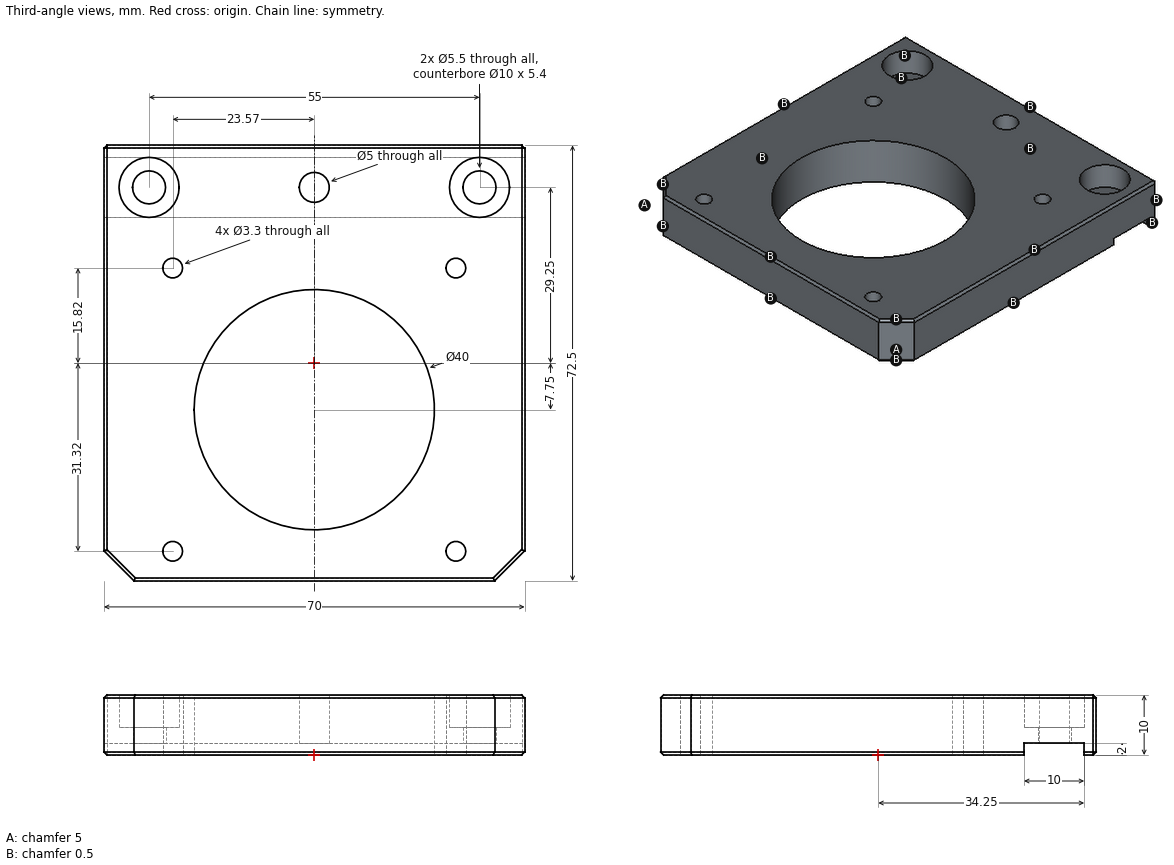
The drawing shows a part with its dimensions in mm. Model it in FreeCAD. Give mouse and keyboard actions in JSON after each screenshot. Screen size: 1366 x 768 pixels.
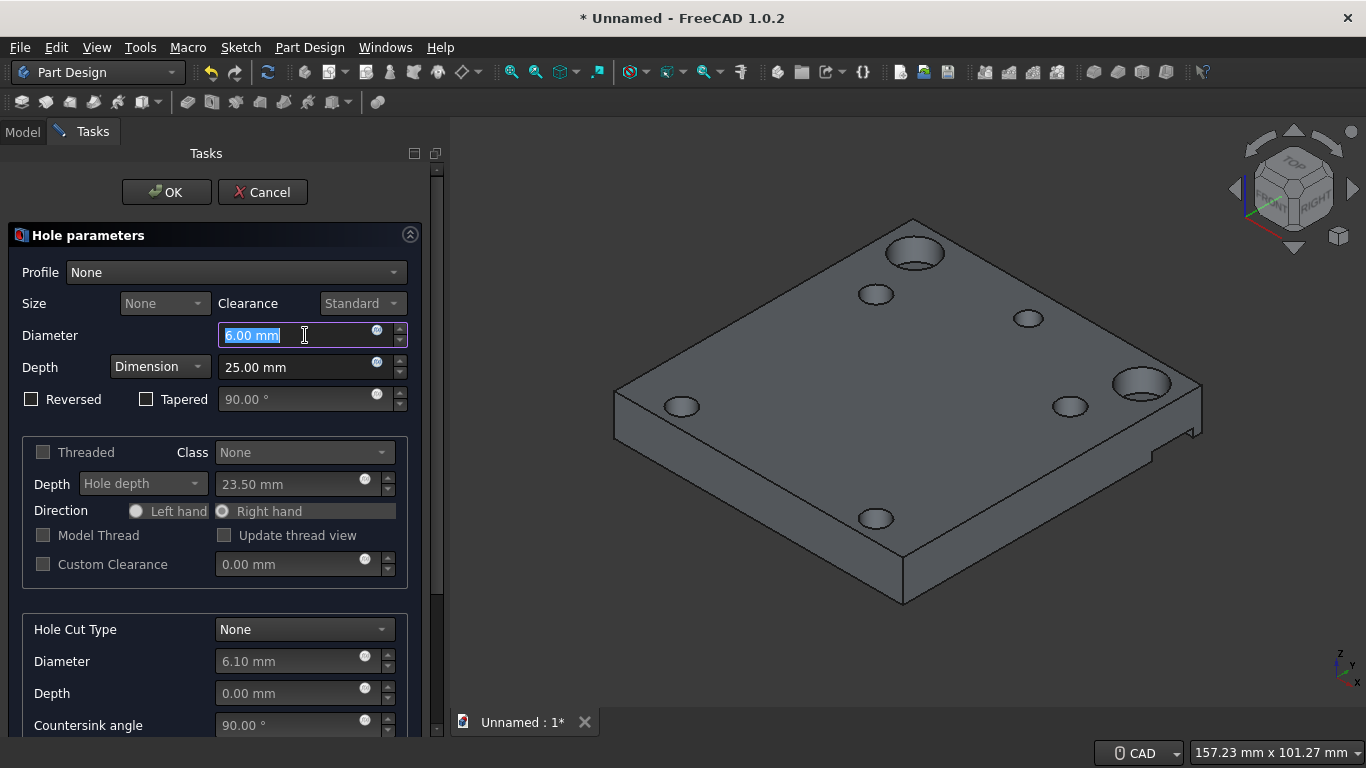
{"action": "type", "text": "3.3"}
{"action": "key", "text": "Tab"}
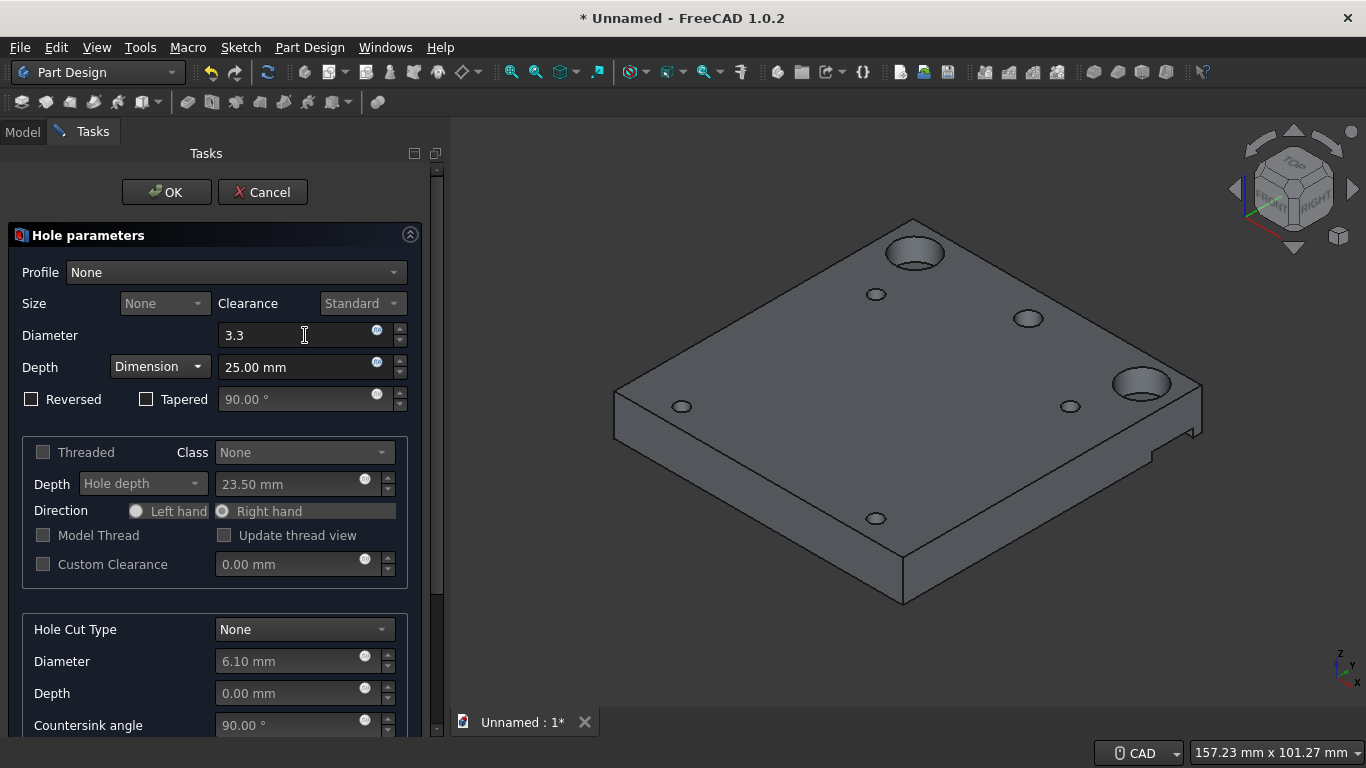
{"action": "left_click", "coordinate": [161, 366]}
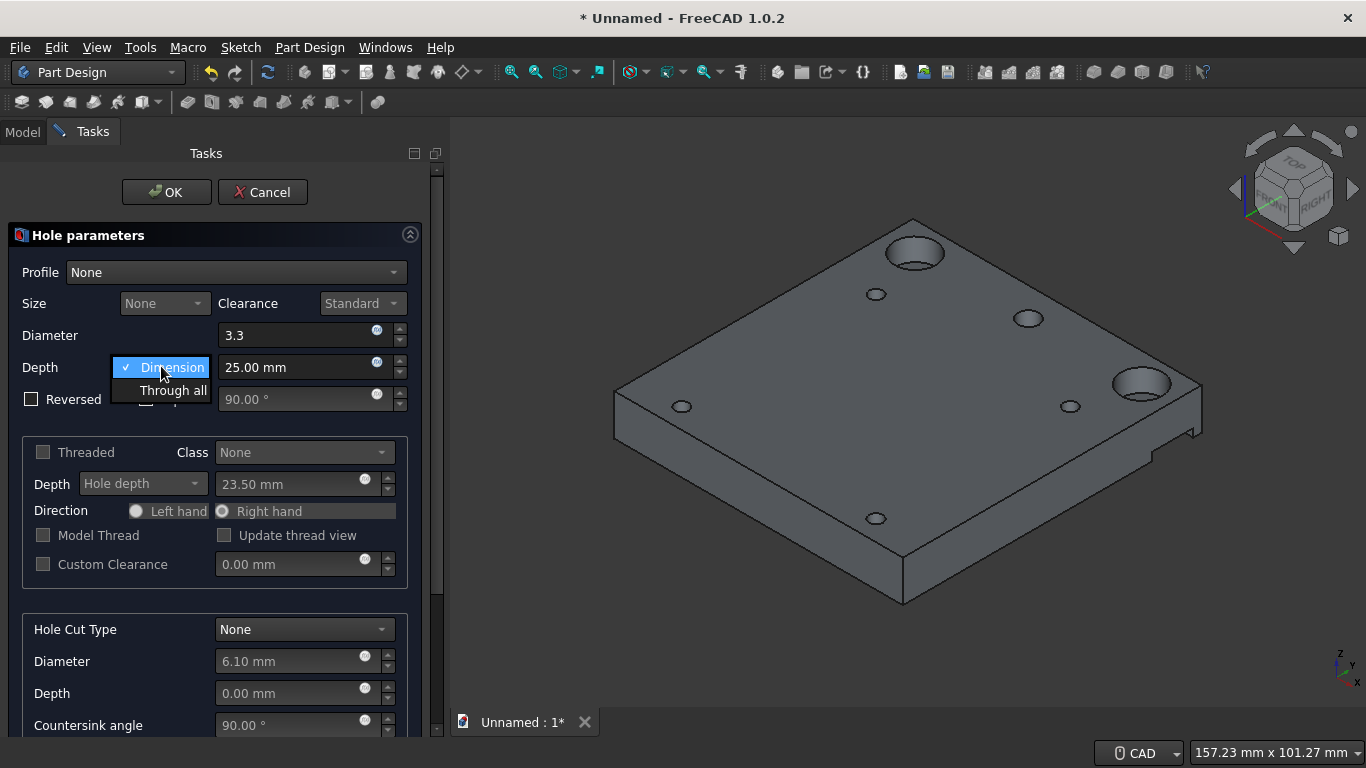
{"action": "left_click", "coordinate": [160, 390]}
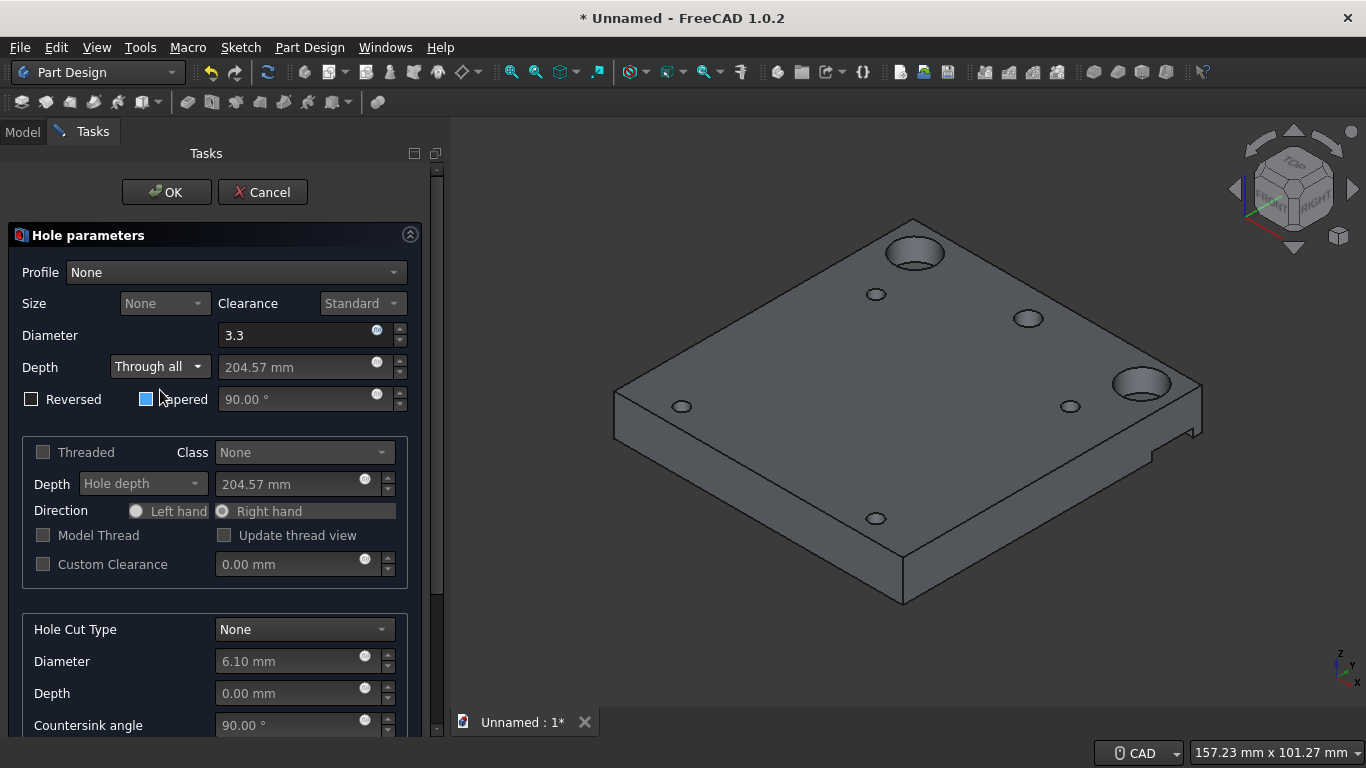
{"action": "left_click", "coordinate": [167, 192]}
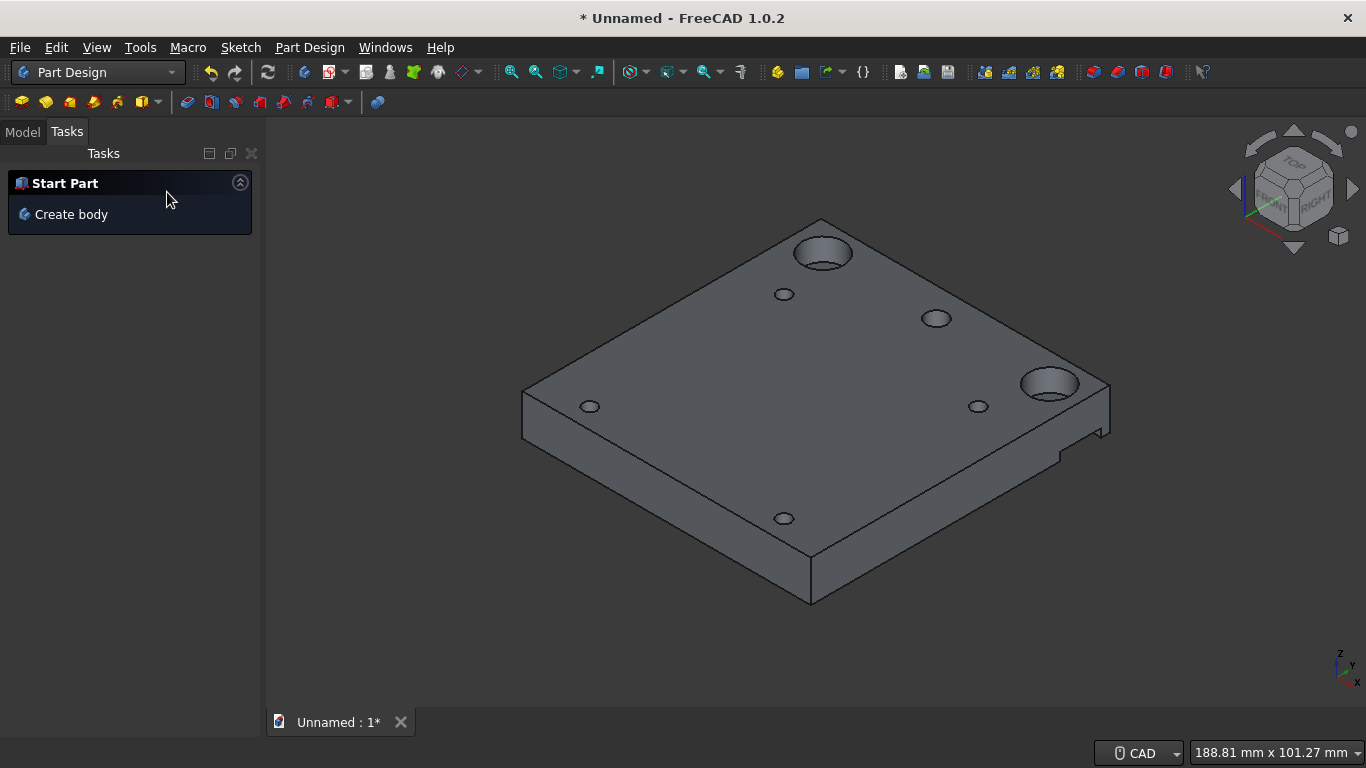
{"action": "left_click", "coordinate": [330, 72]}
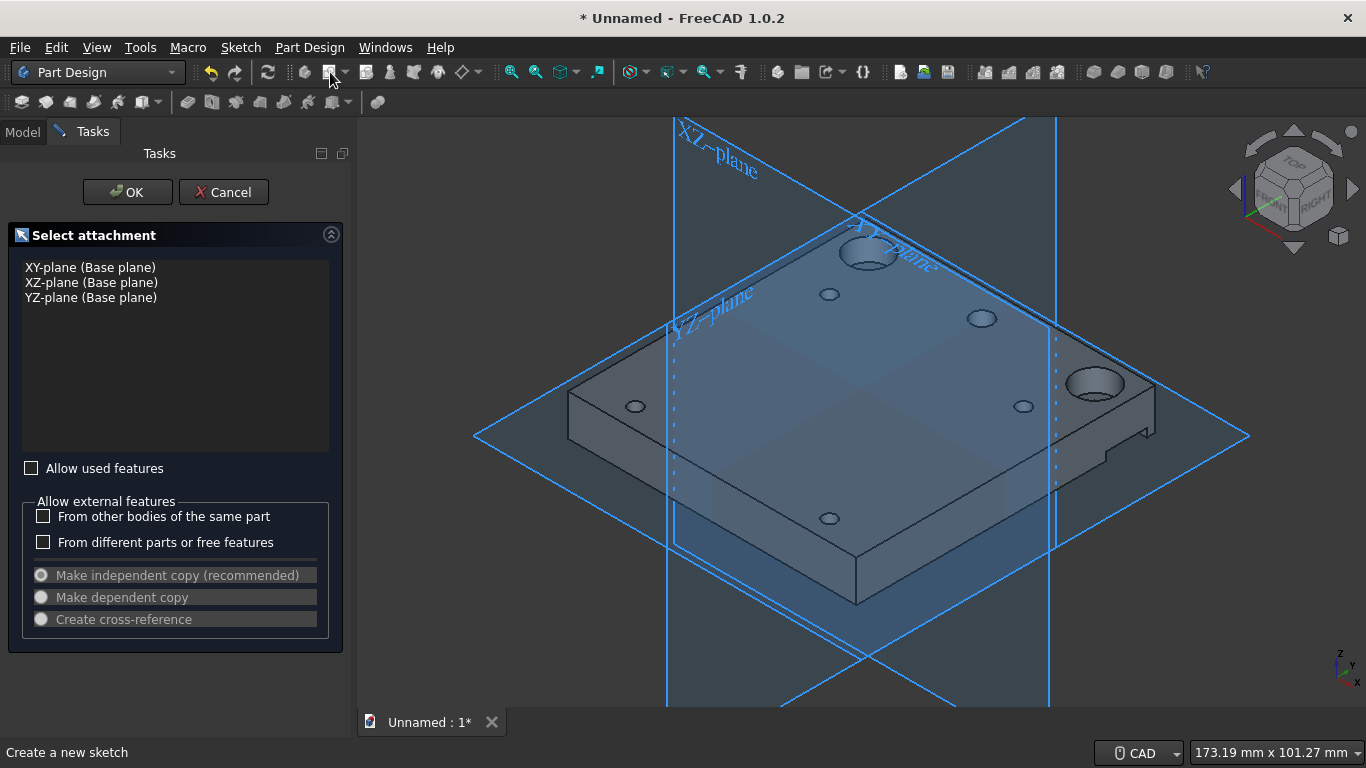
{"action": "left_click", "coordinate": [82, 268]}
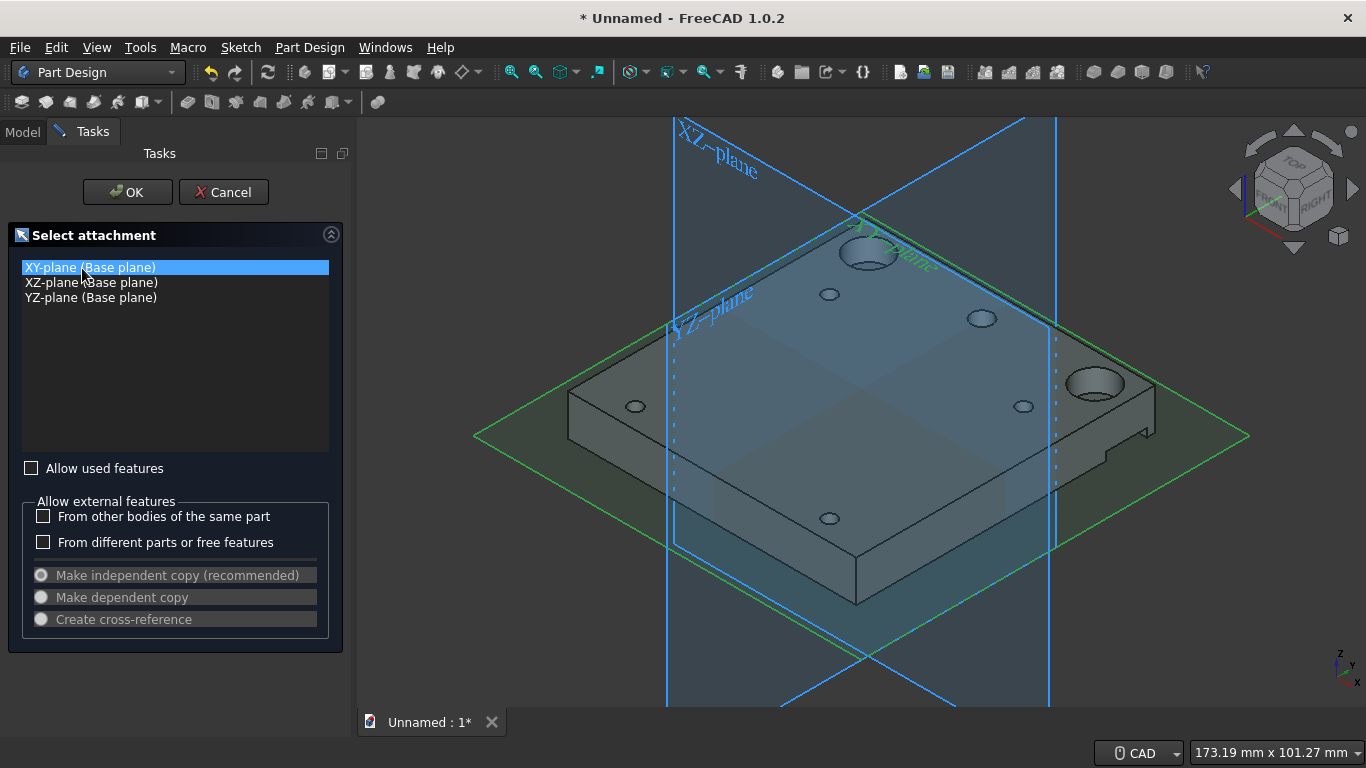
{"action": "left_click", "coordinate": [128, 192]}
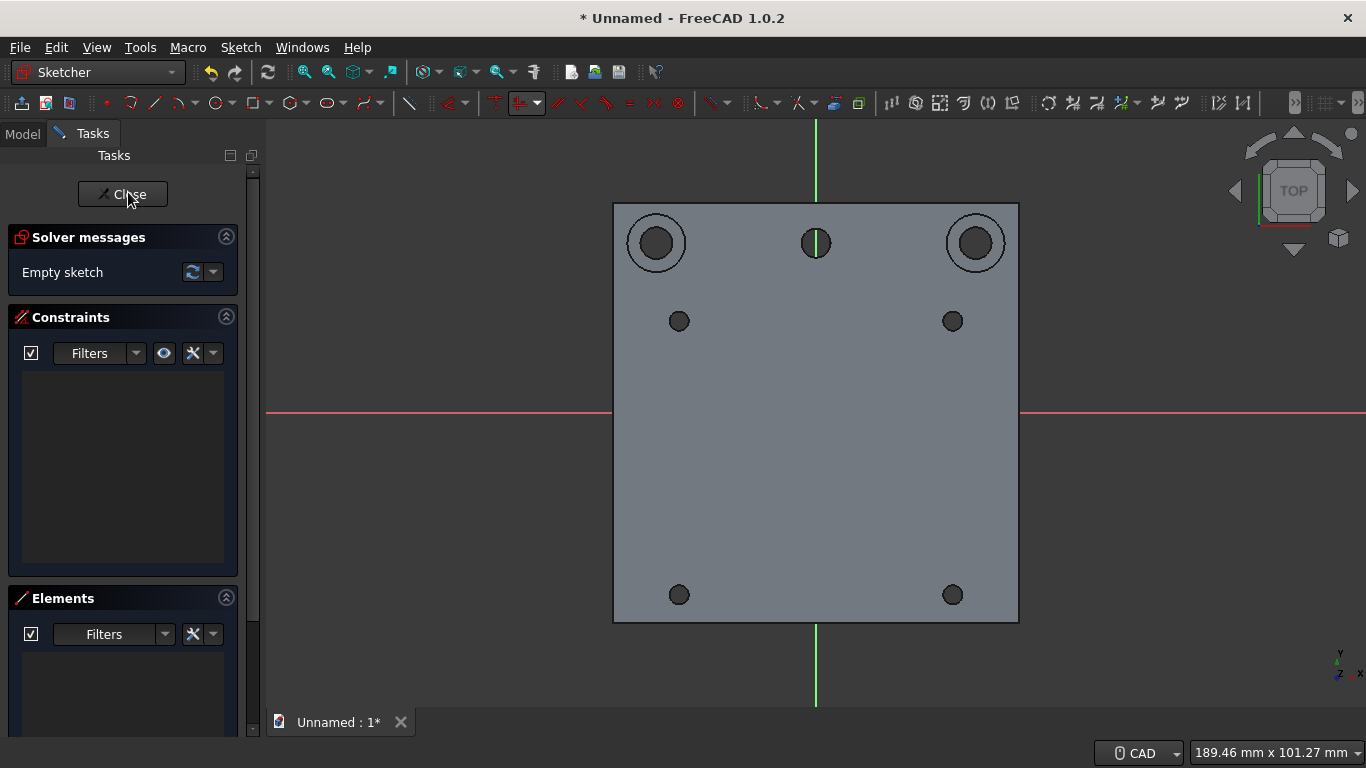
{"action": "left_click", "coordinate": [70, 104]}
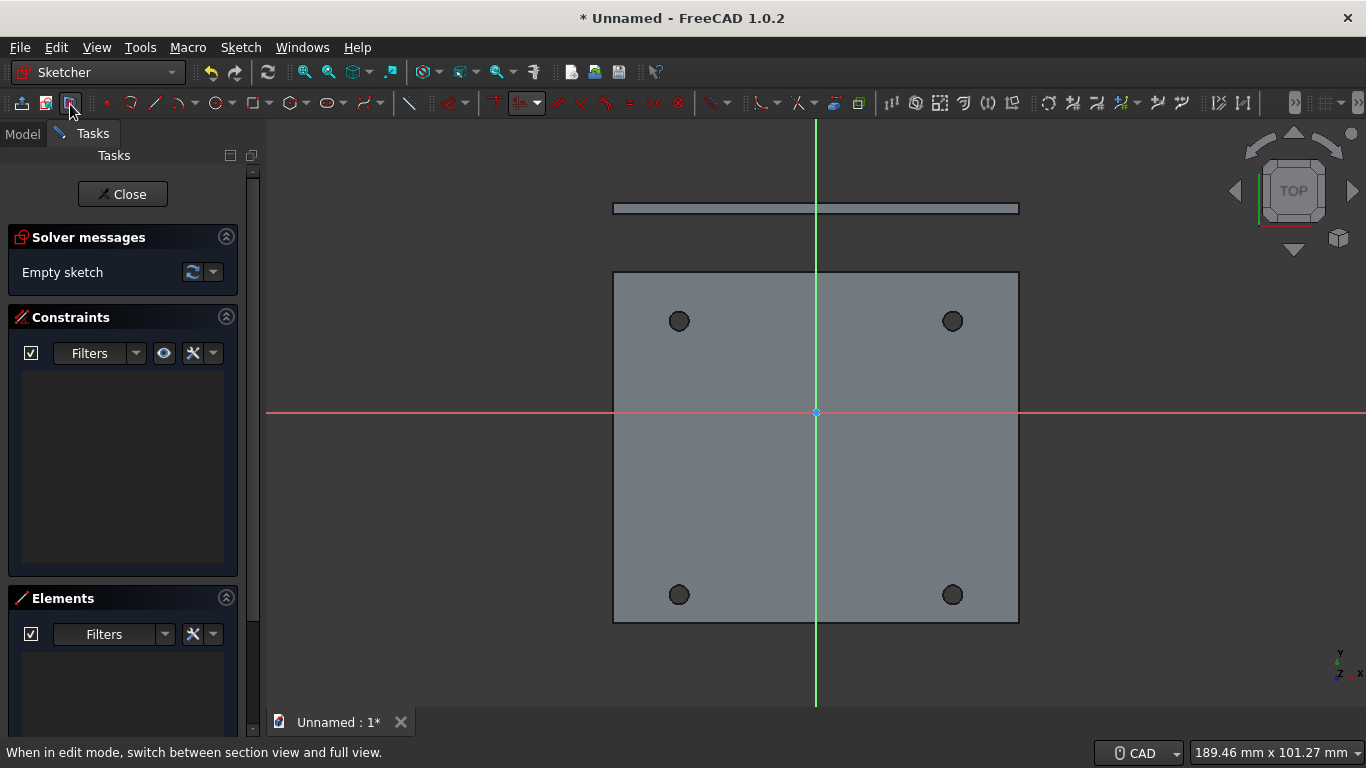
{"action": "scroll", "coordinate": [955, 549], "scroll_direction": "up", "scroll_amount": 2}